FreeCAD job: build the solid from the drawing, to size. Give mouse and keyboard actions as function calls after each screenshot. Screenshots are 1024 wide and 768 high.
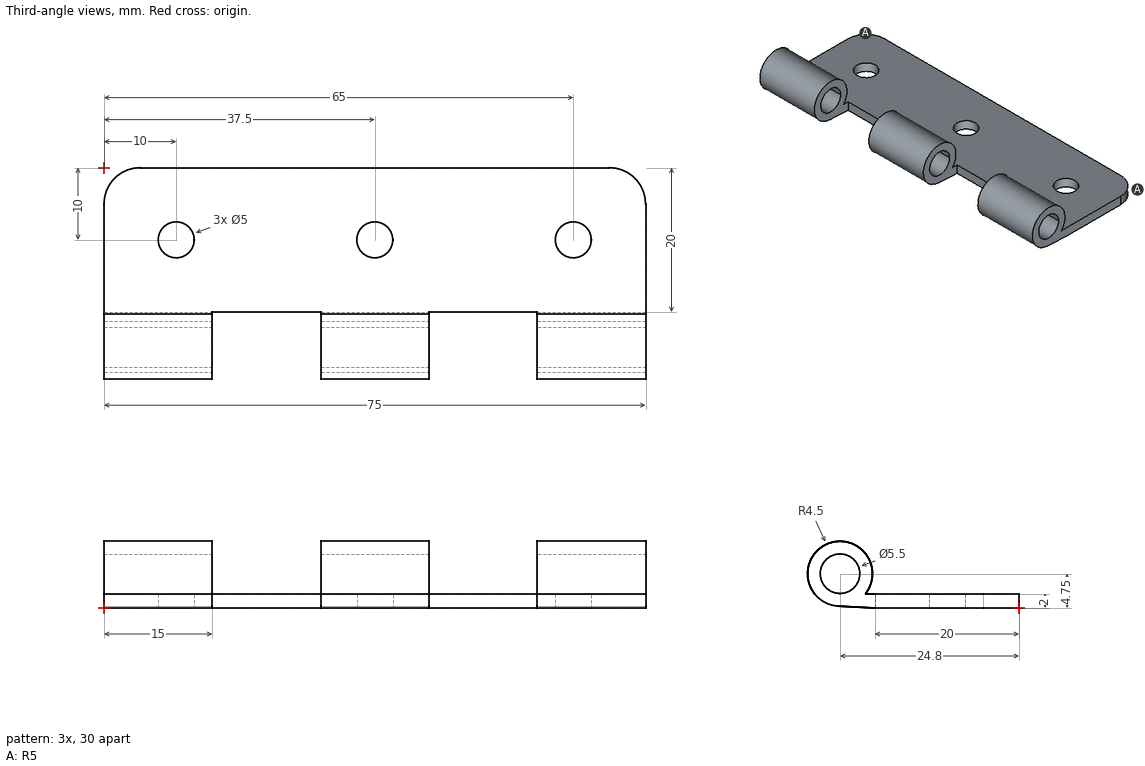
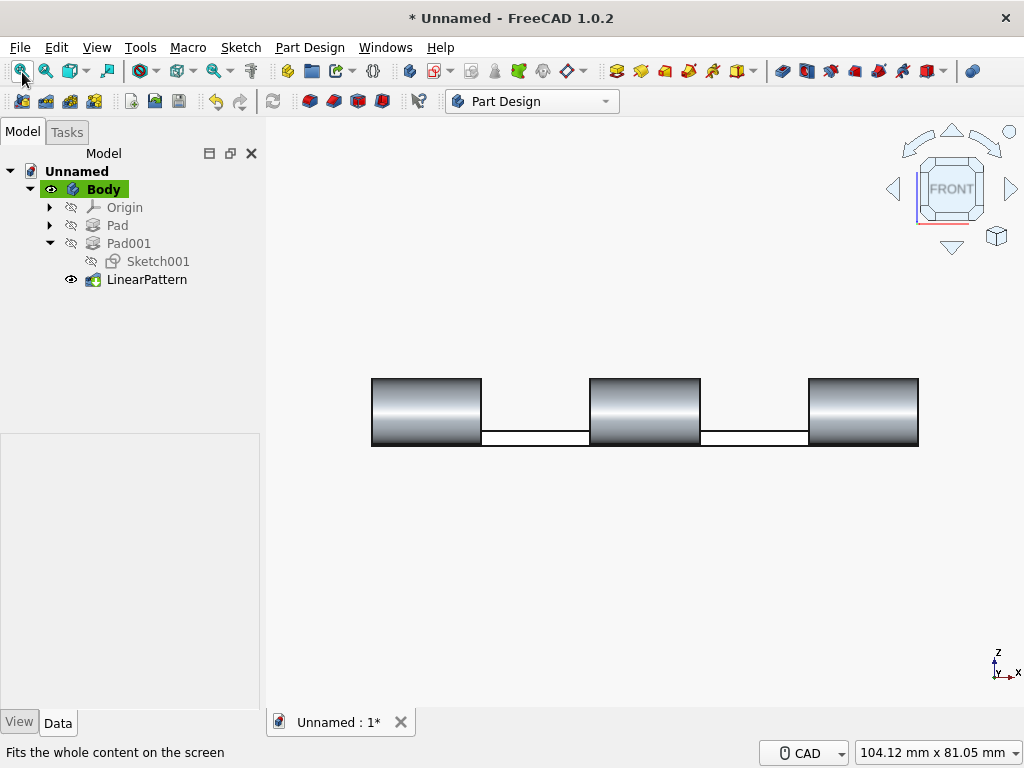
key(0)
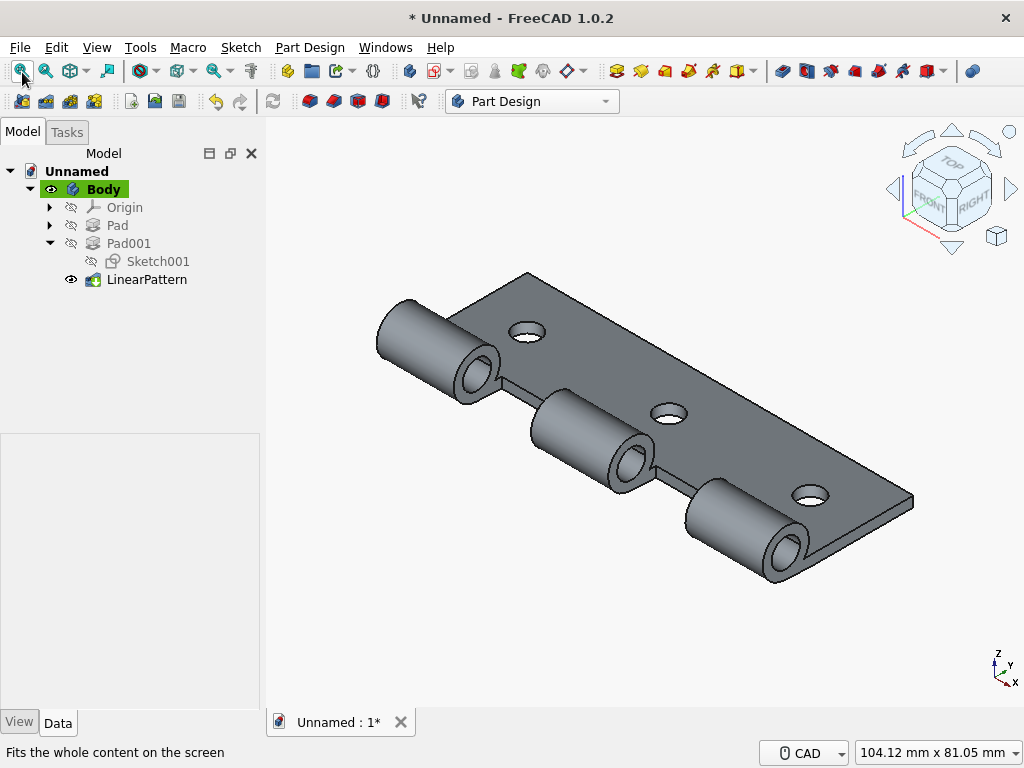
scroll(527, 278, up, 6)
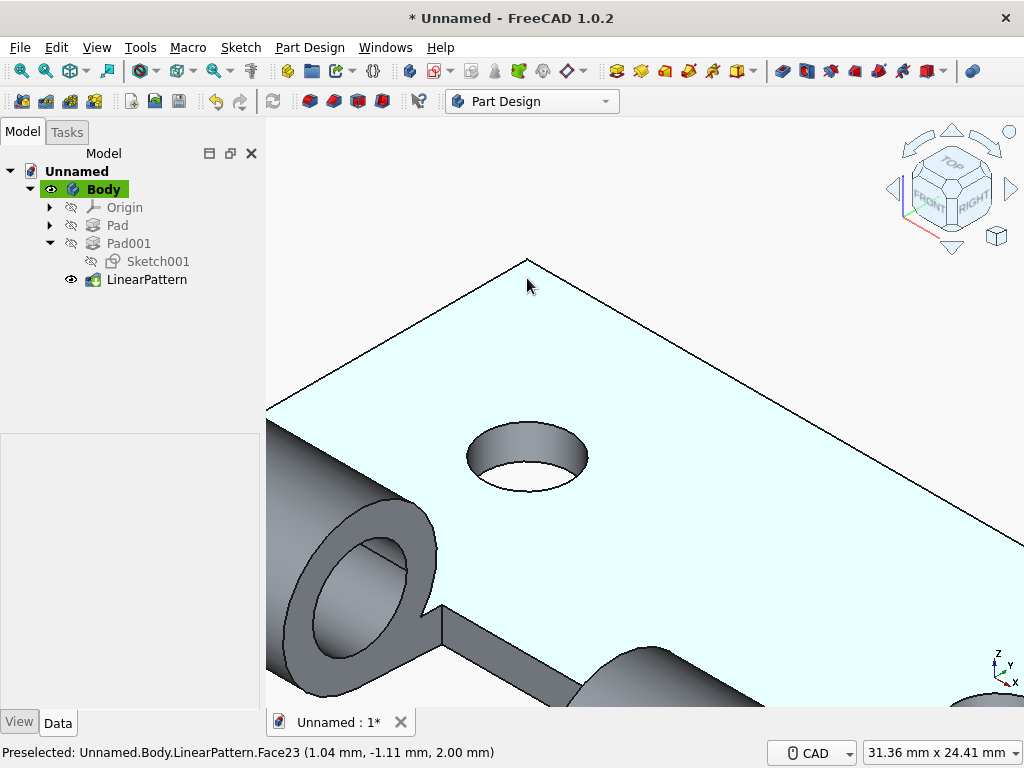
key(v)
key(f)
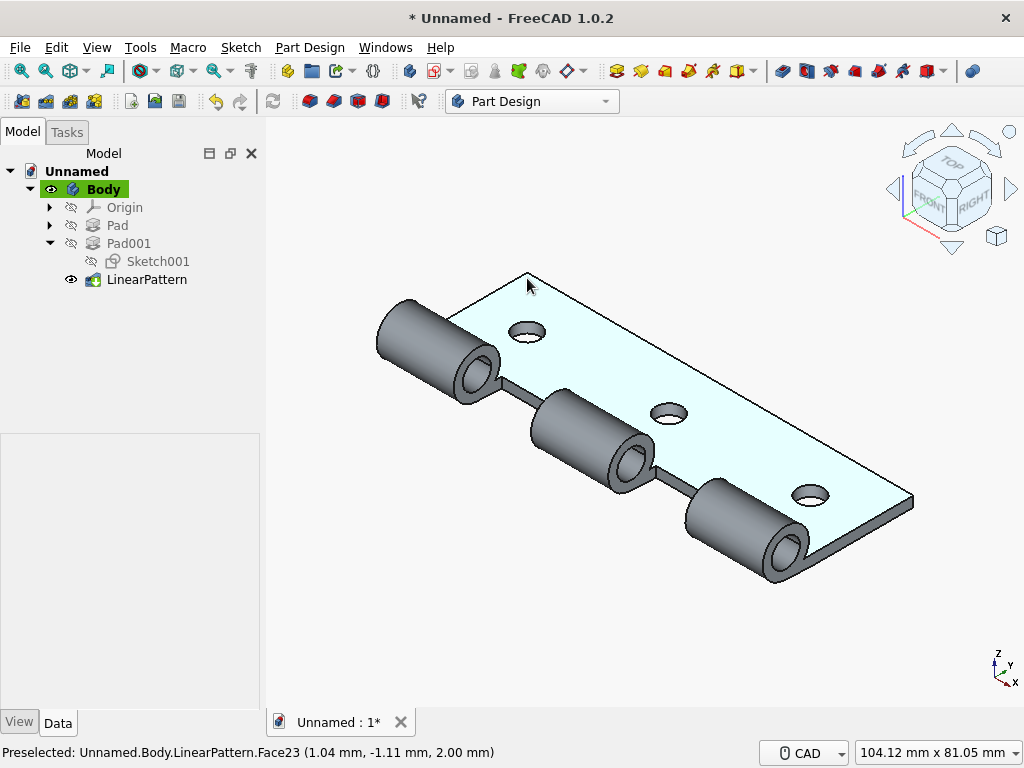
key(2)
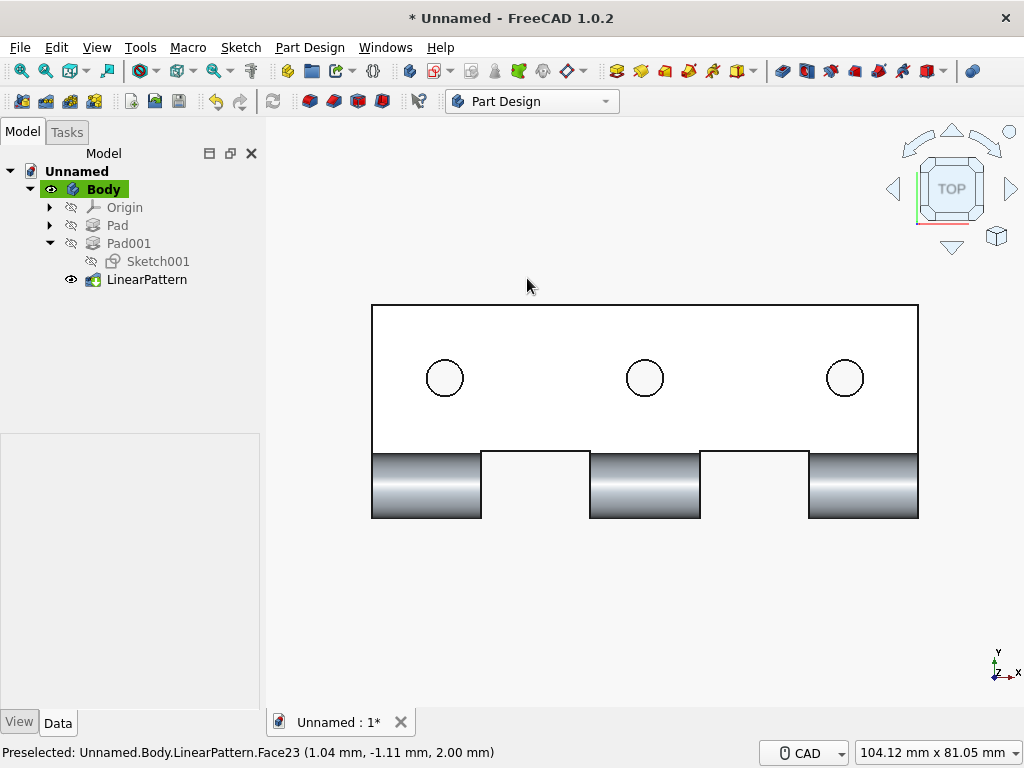
scroll(372, 304, up, 6)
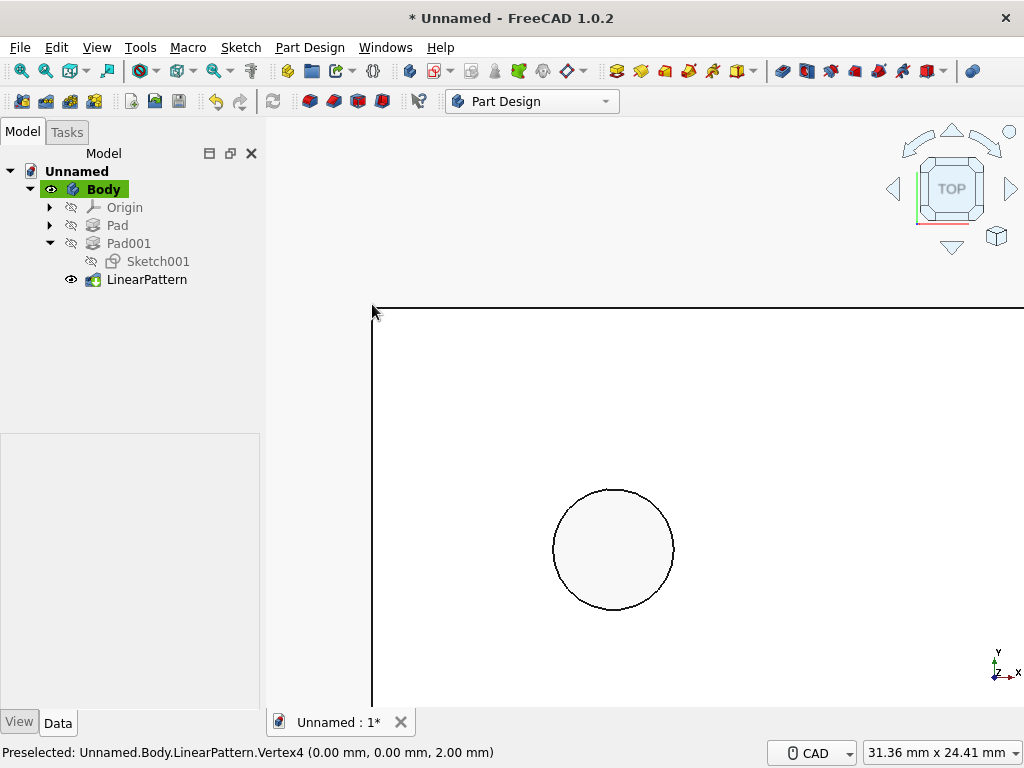
click(22, 72)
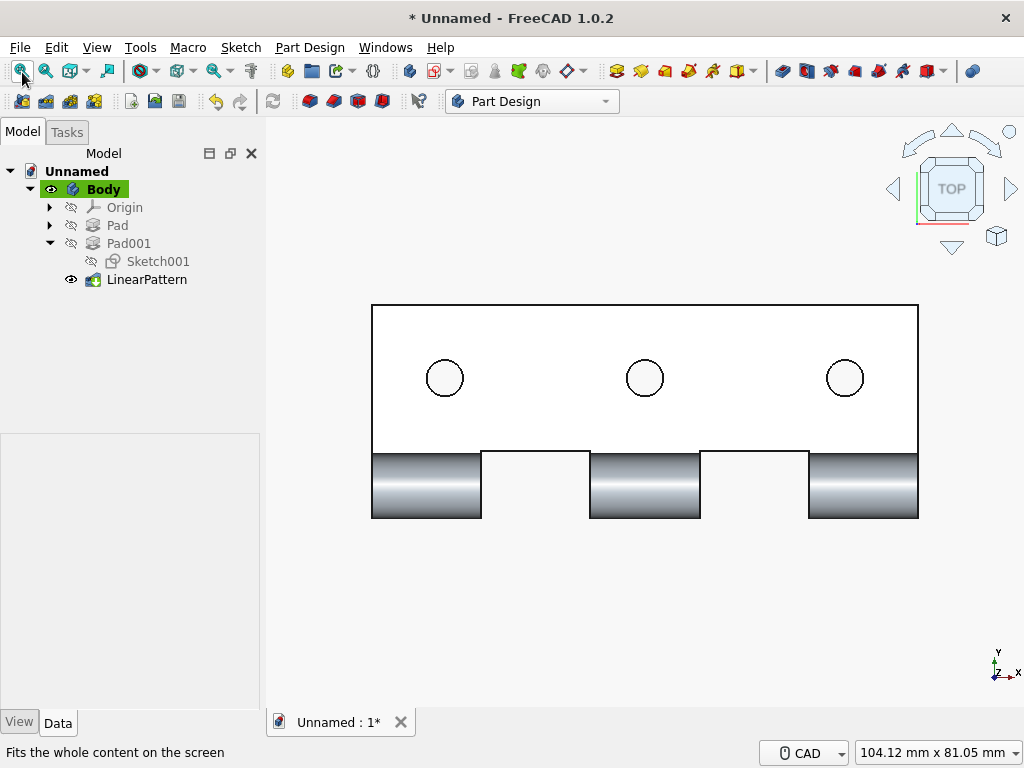
key(1)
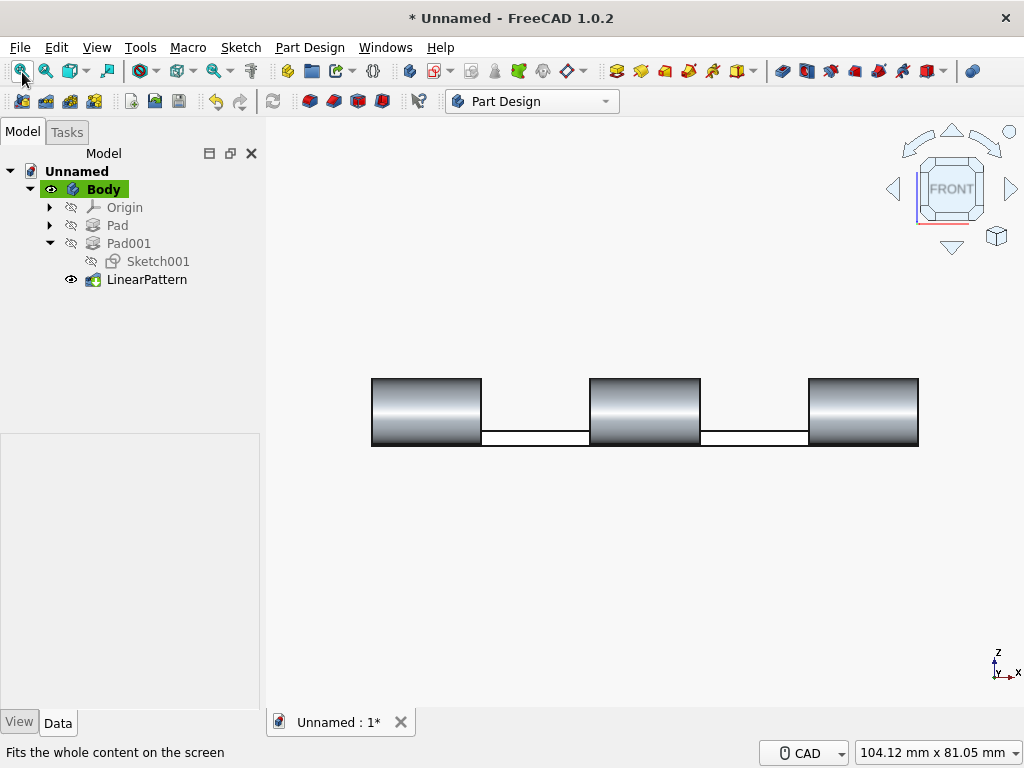
scroll(372, 437, up, 6)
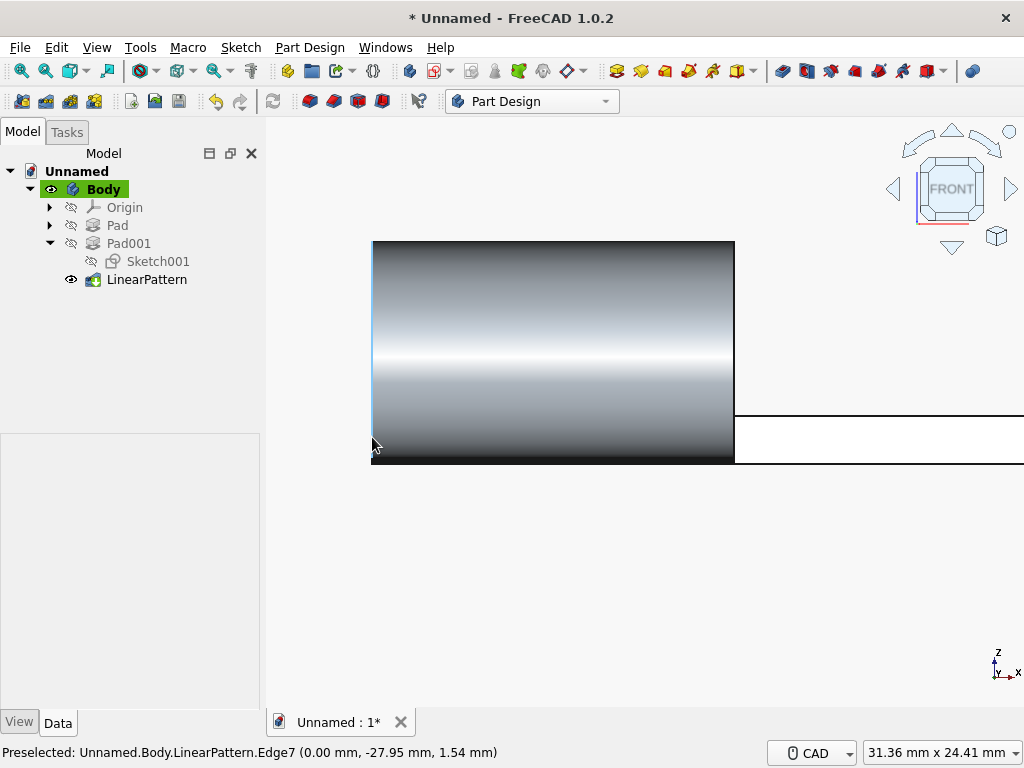
click(22, 72)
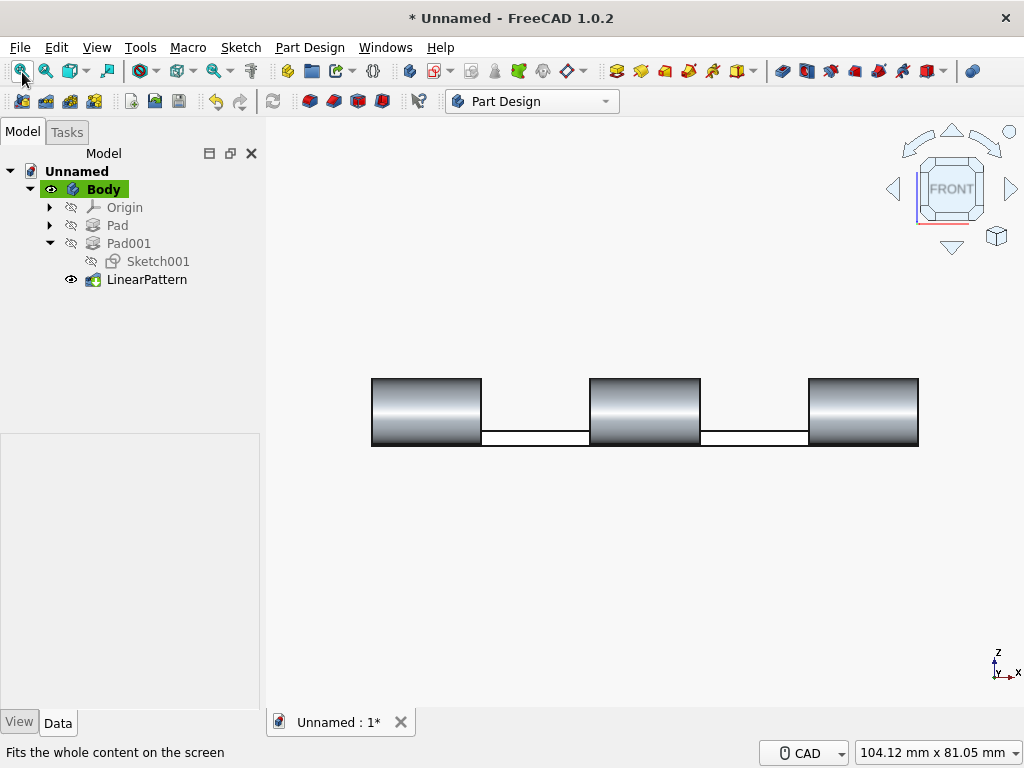
key(3)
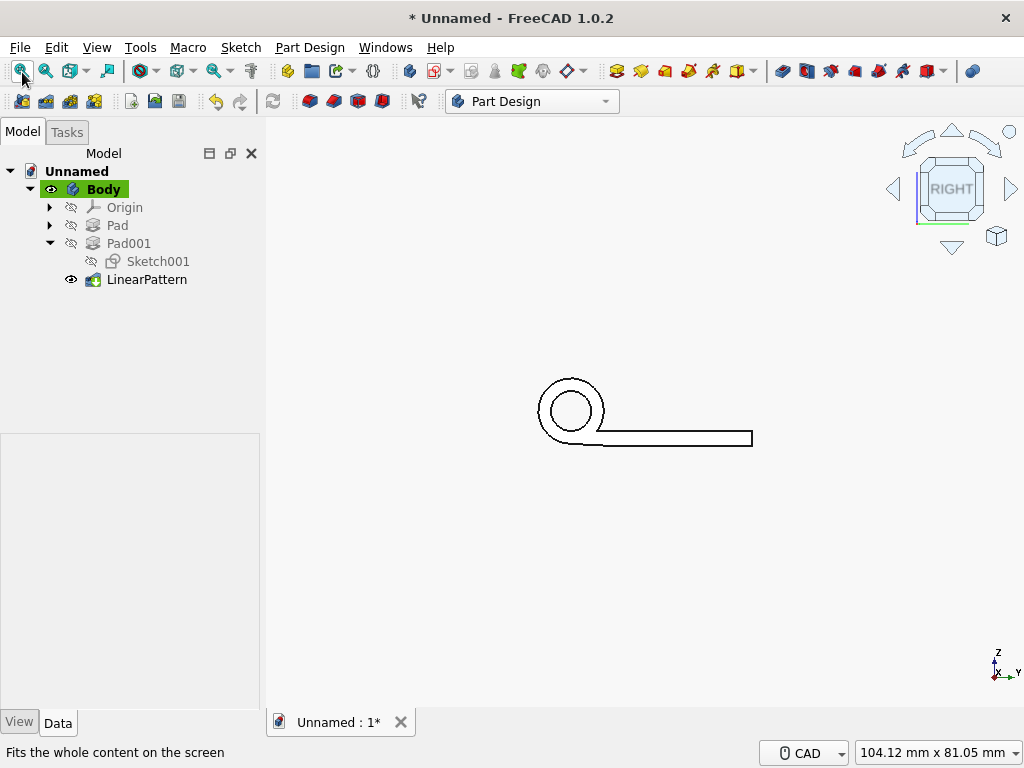
key(v)
key(f)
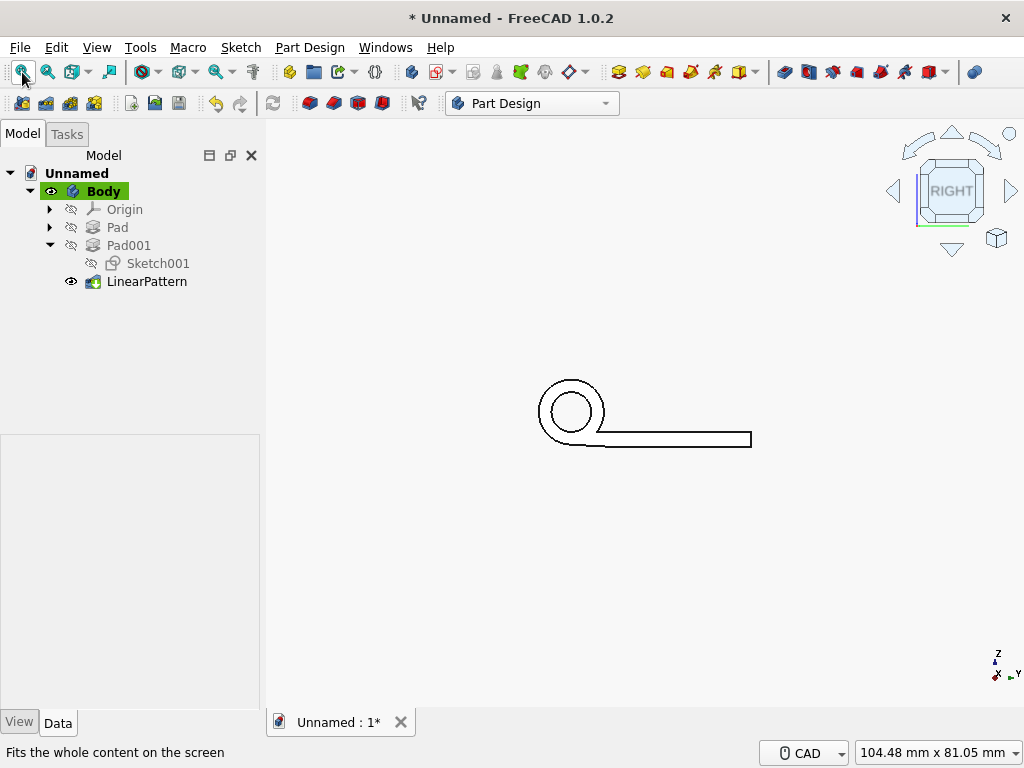
click(751, 438)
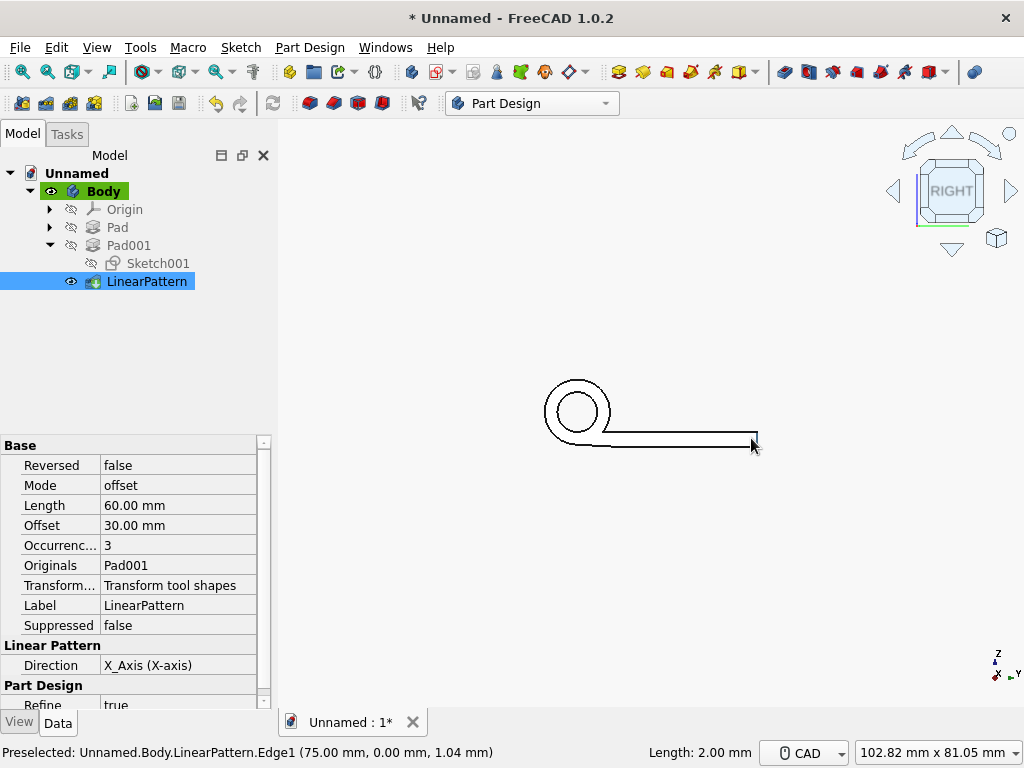
scroll(757, 438, up, 6)